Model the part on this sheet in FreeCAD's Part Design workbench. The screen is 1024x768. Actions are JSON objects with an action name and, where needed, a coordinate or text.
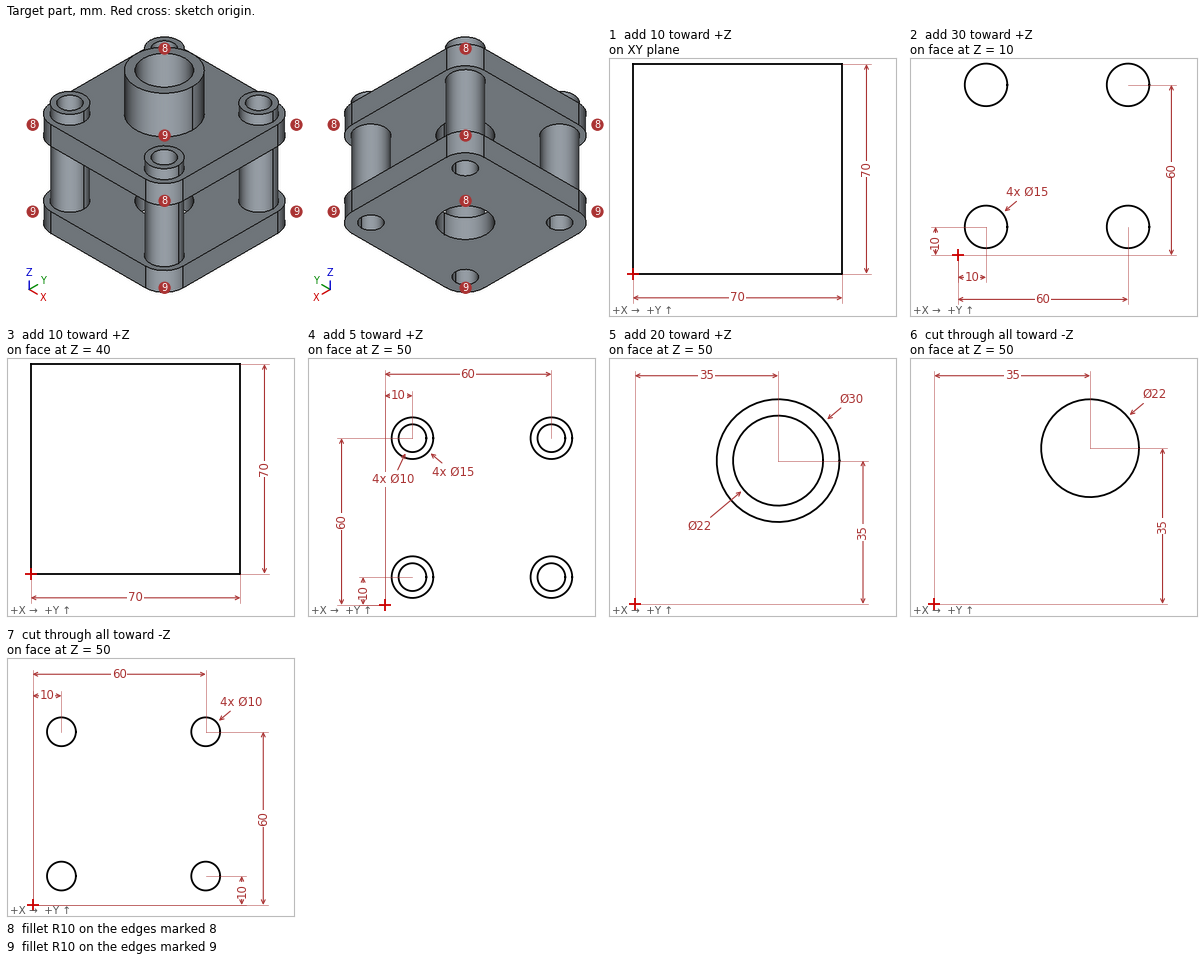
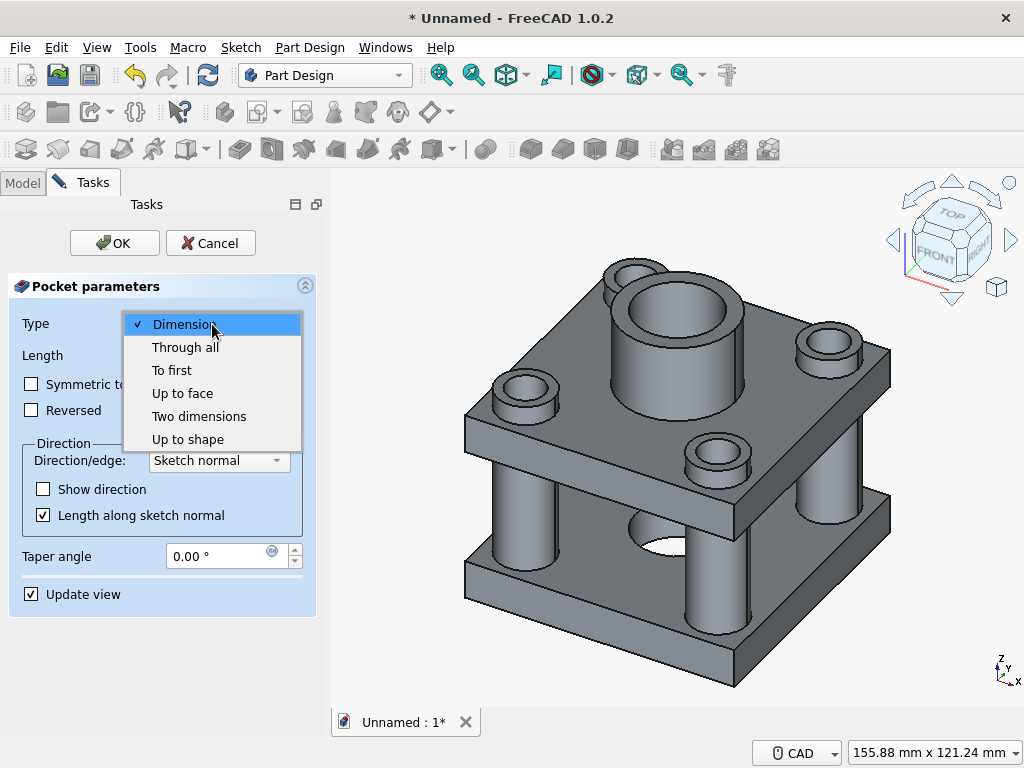
{"action": "left_click", "coordinate": [212, 348]}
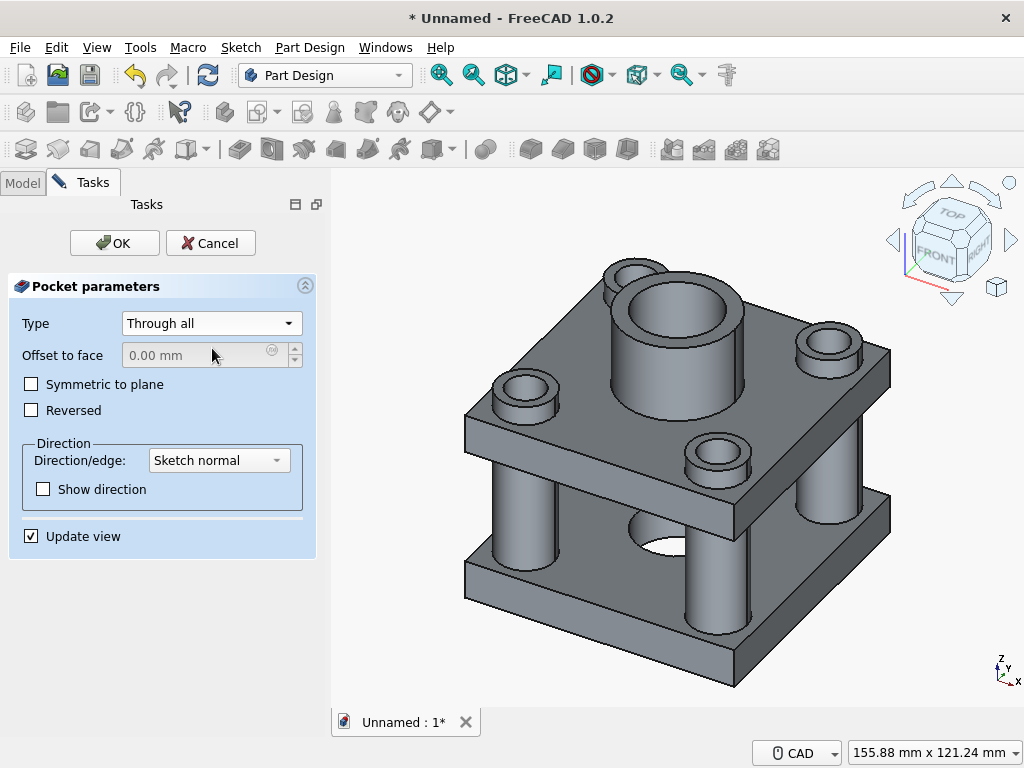
{"action": "left_click", "coordinate": [115, 243]}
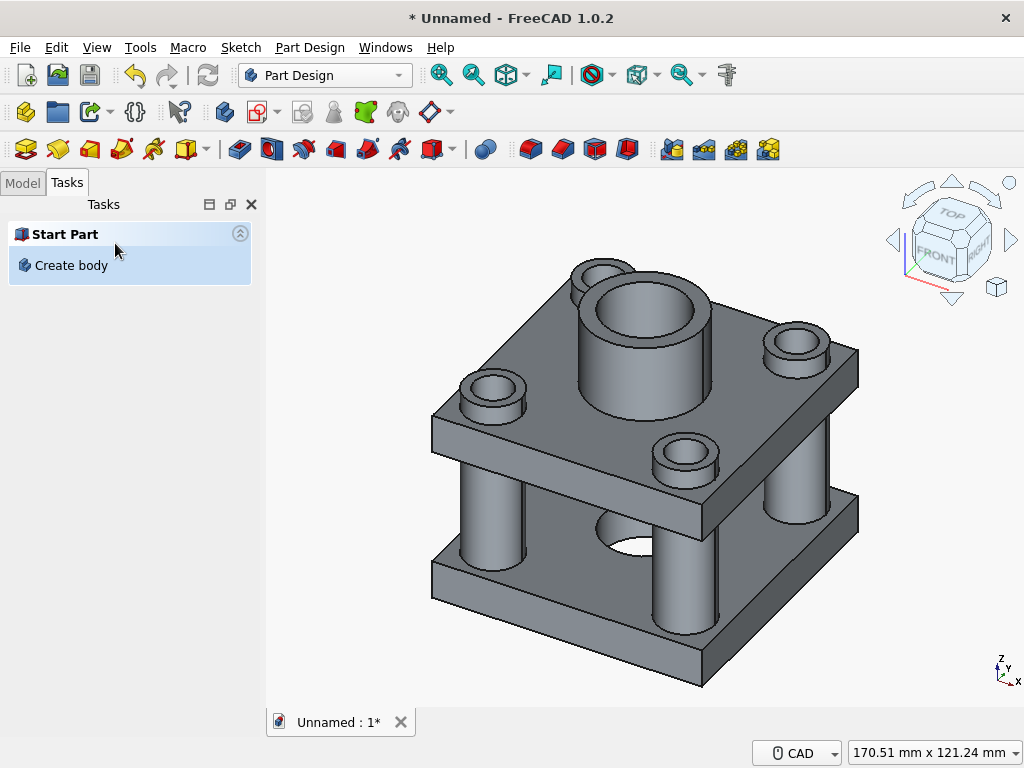
{"action": "left_click", "coordinate": [702, 522]}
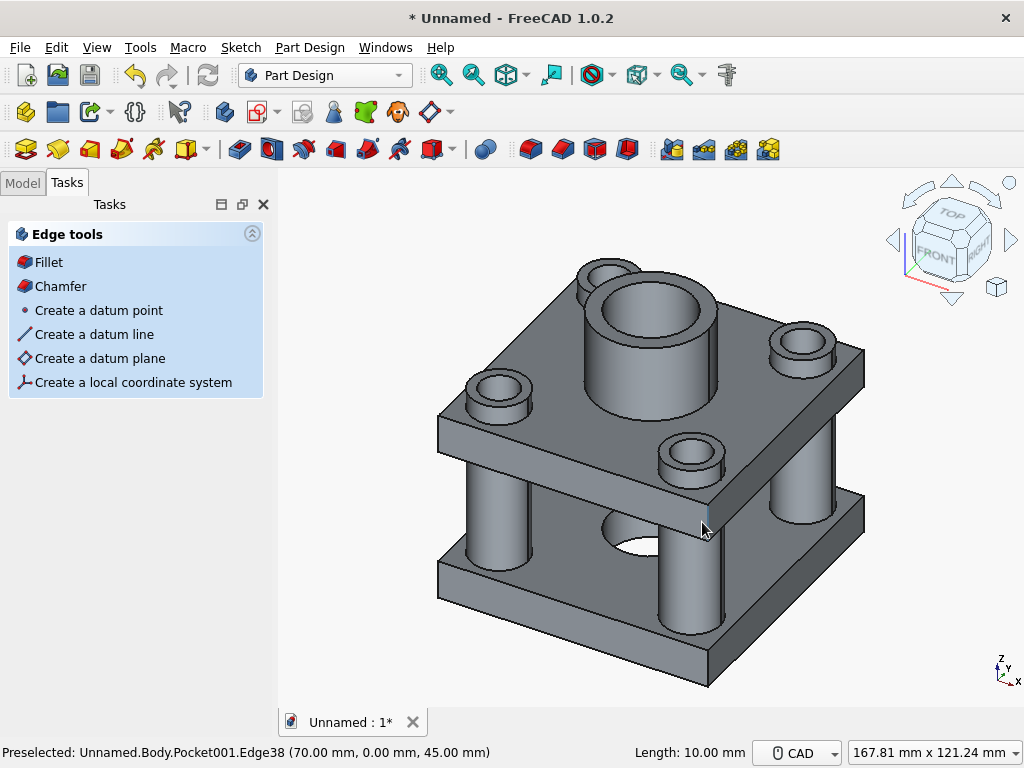
{"action": "key", "text": "0"}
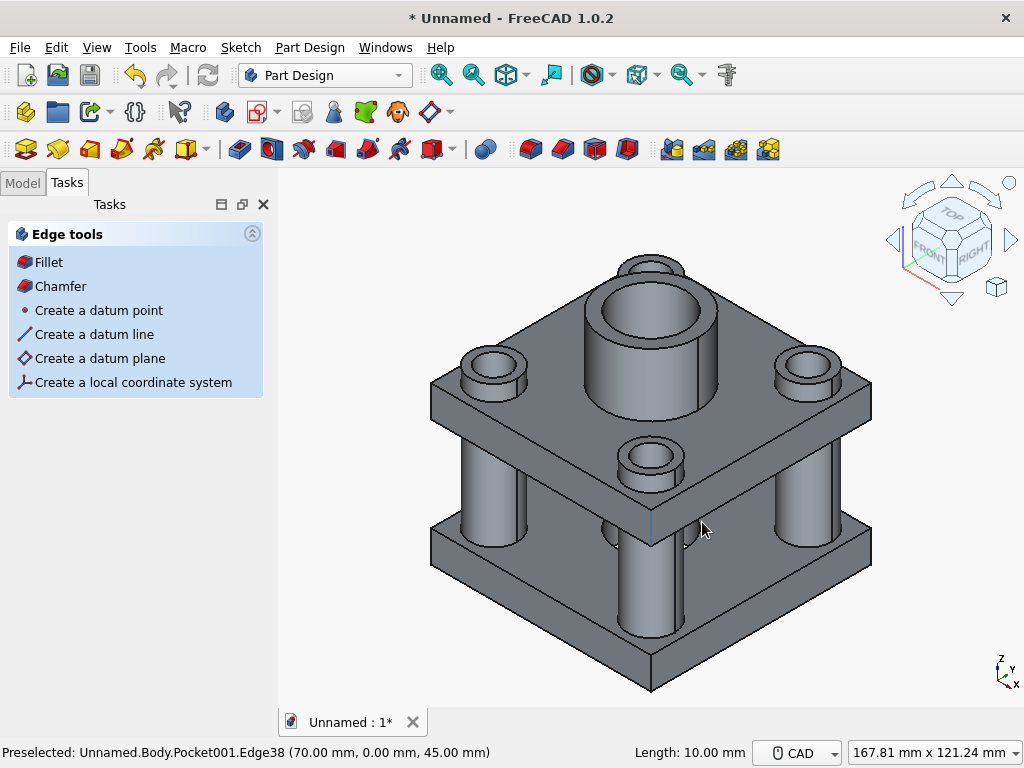
{"action": "key", "text": "2"}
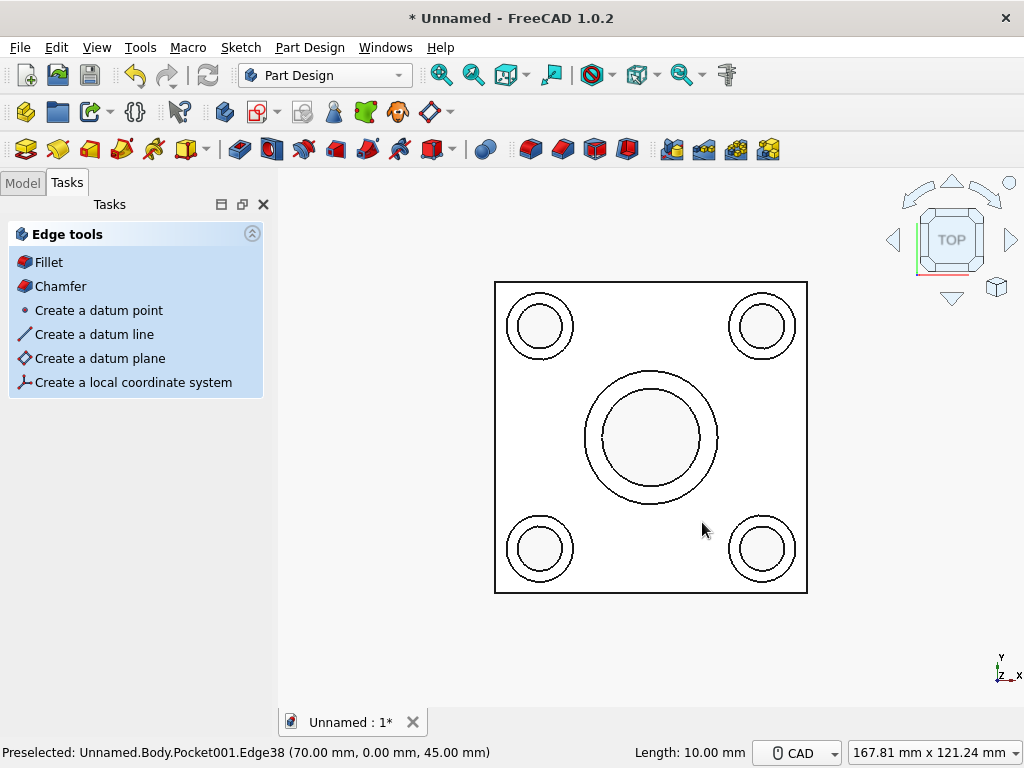
{"action": "key", "text": "1"}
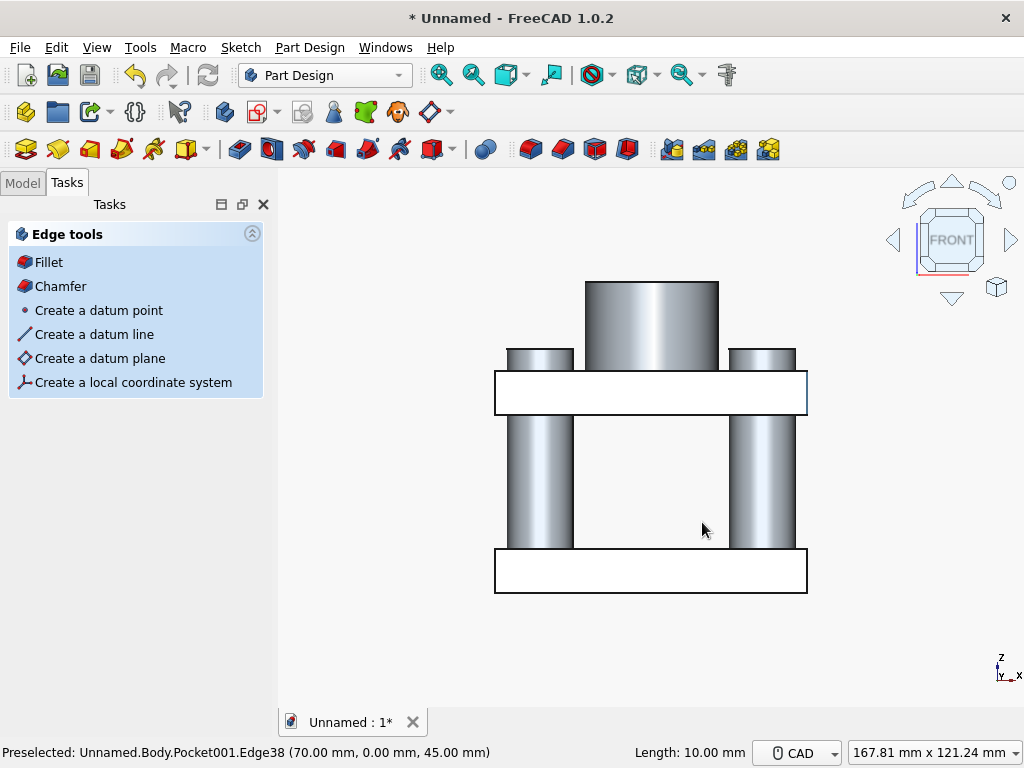
{"action": "left_click", "coordinate": [495, 392], "text": "ctrl"}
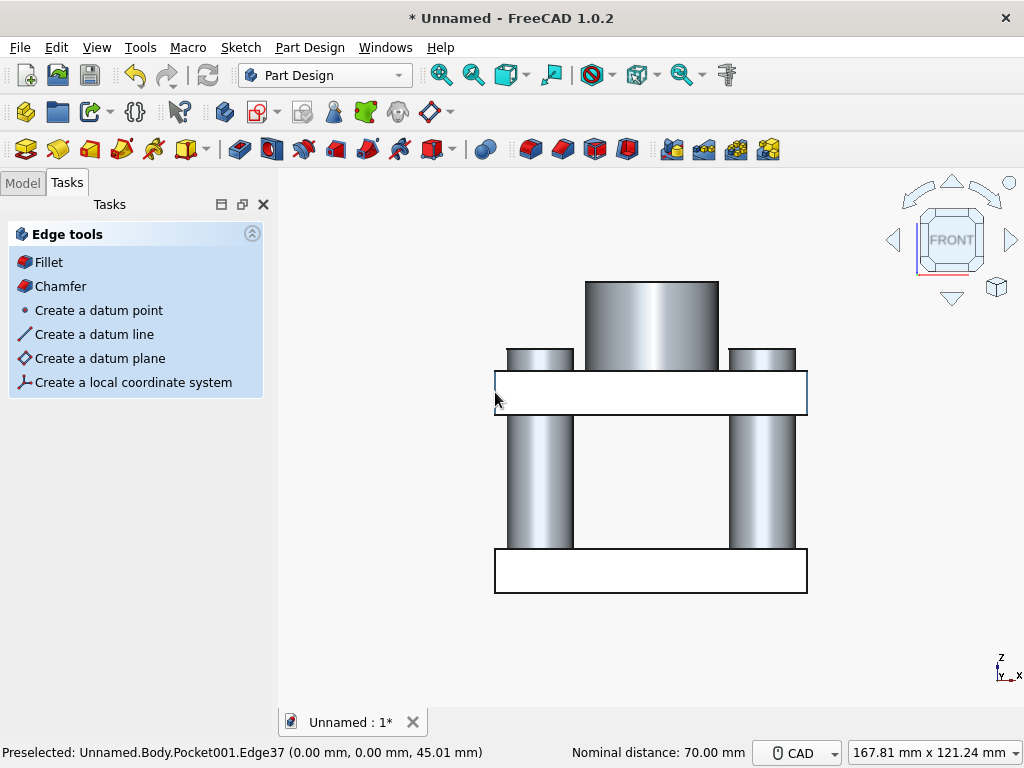
{"action": "key", "text": "3"}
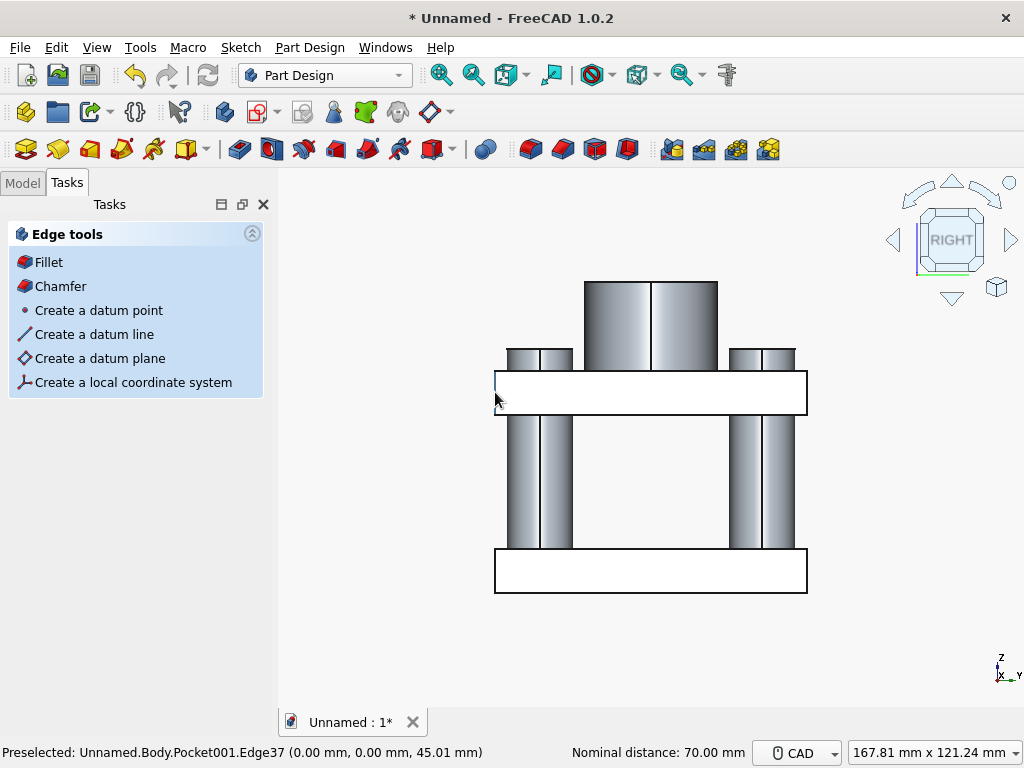
{"action": "left_click", "coordinate": [807, 392], "text": "ctrl"}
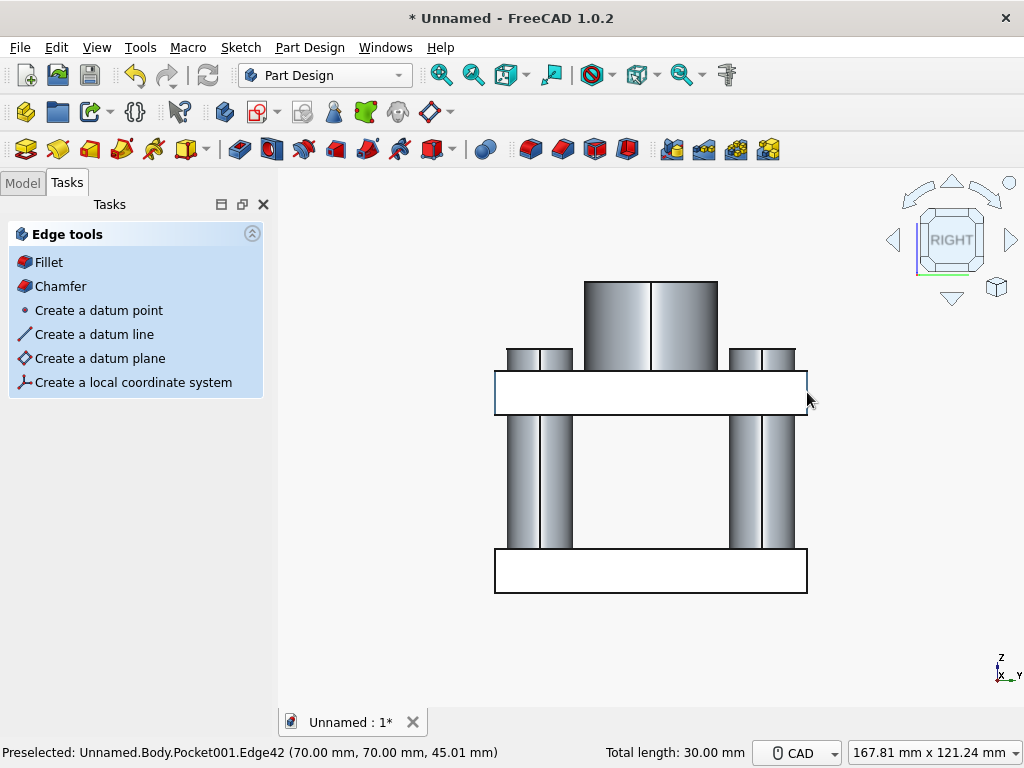
{"action": "key", "text": "5"}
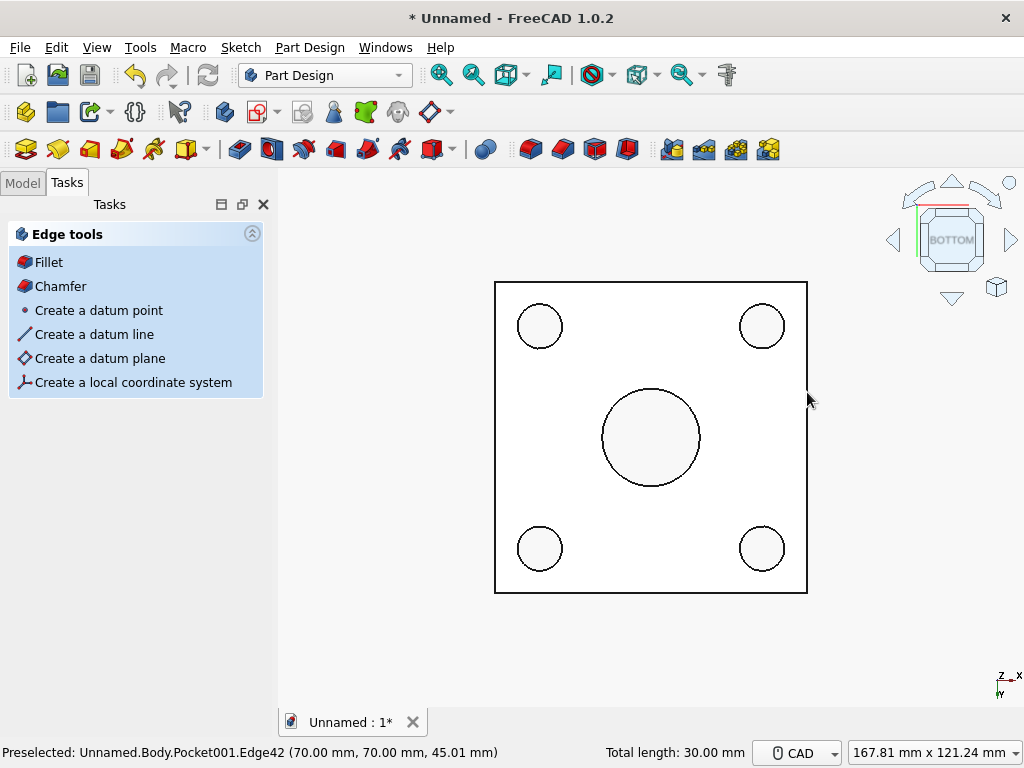
{"action": "key", "text": "4"}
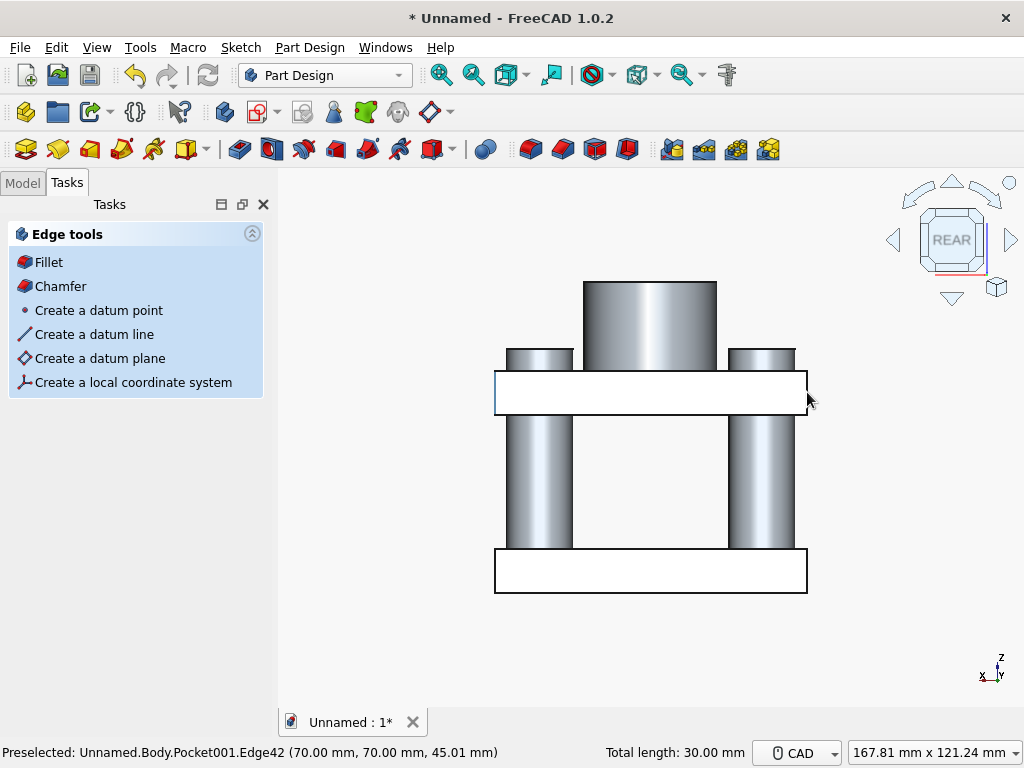
{"action": "left_click", "coordinate": [807, 392], "text": "ctrl"}